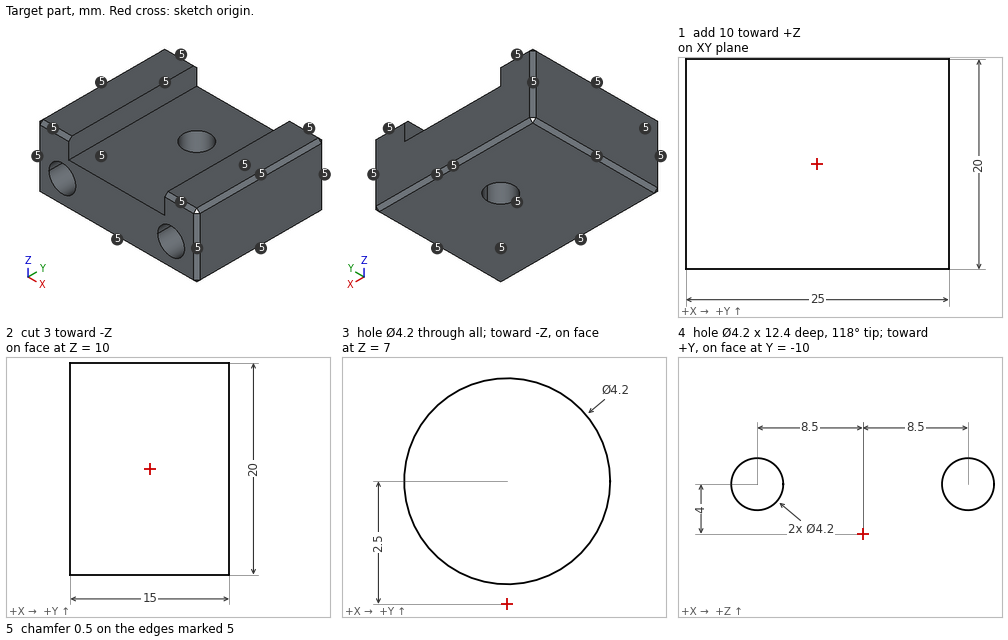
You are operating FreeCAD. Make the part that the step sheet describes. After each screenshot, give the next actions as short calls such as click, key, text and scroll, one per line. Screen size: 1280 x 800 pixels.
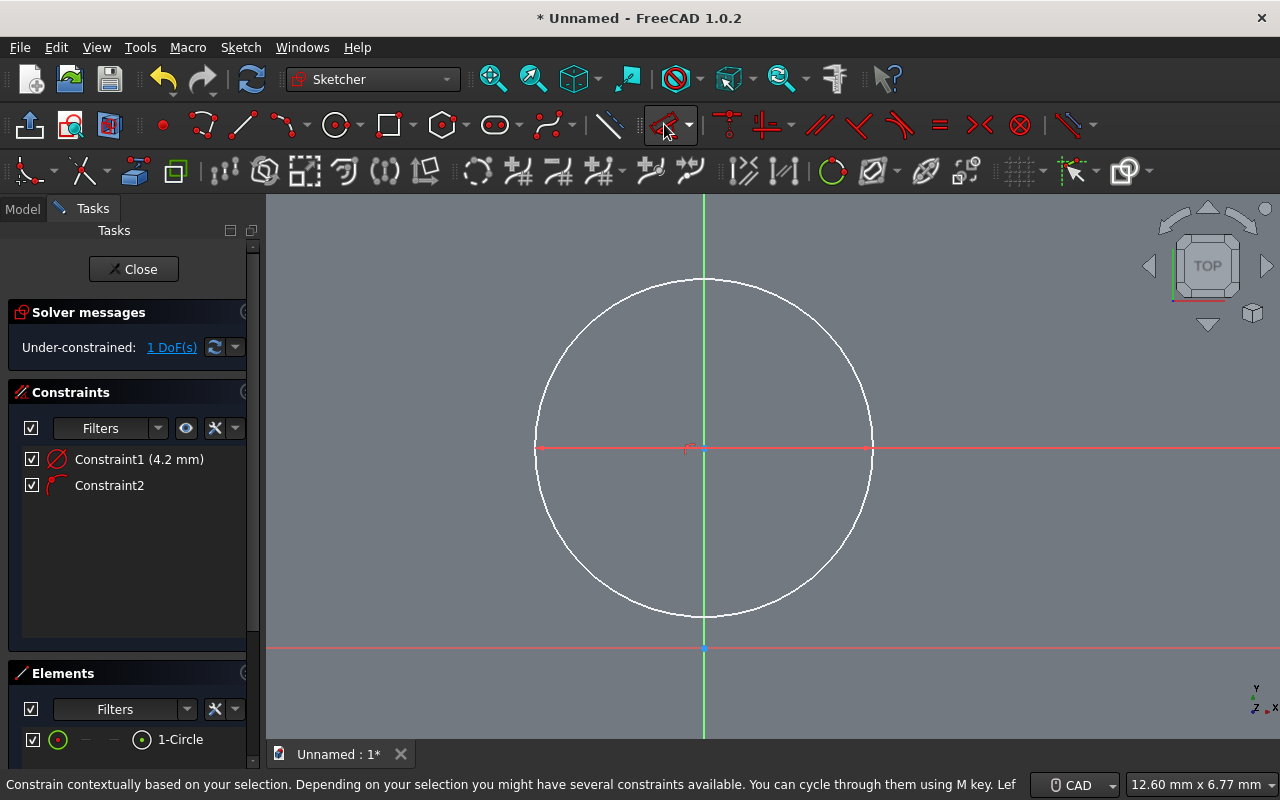
click(704, 448)
click(738, 548)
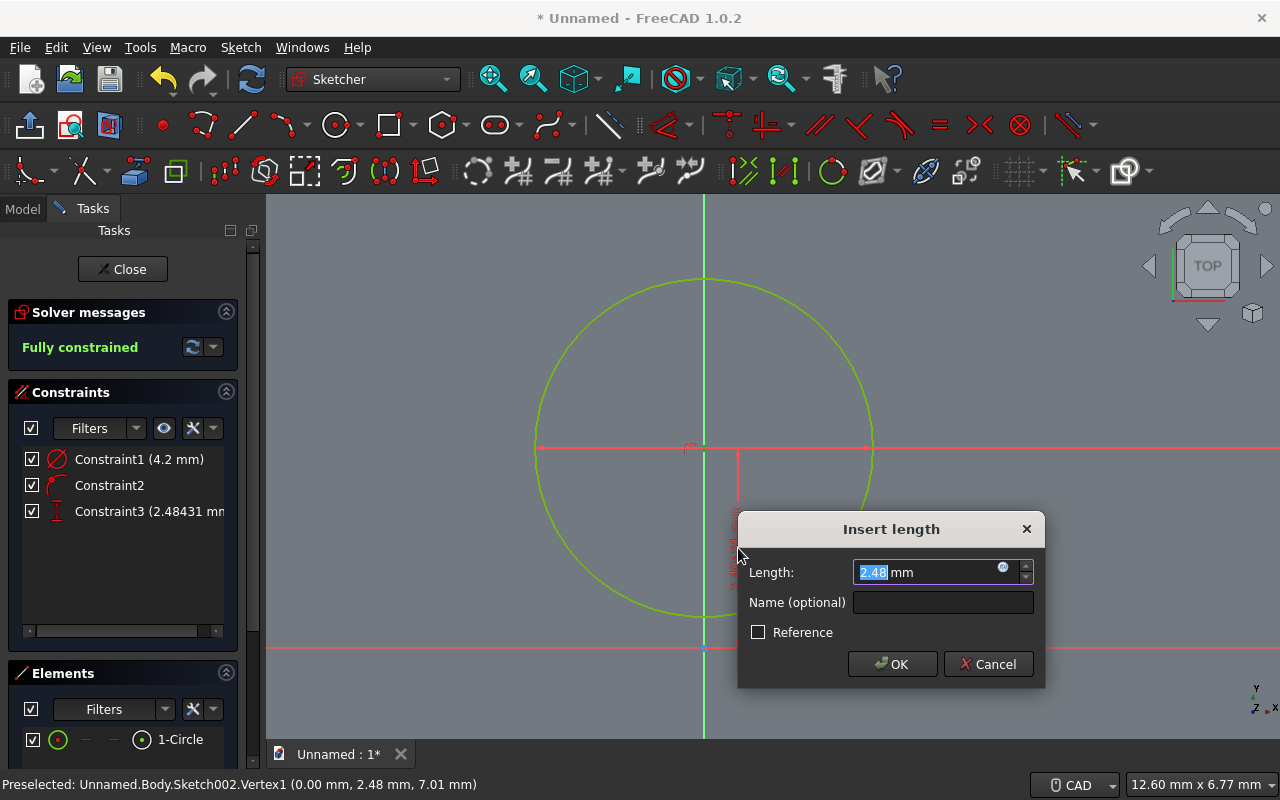
text(2.5)
key(Return)
key(Escape)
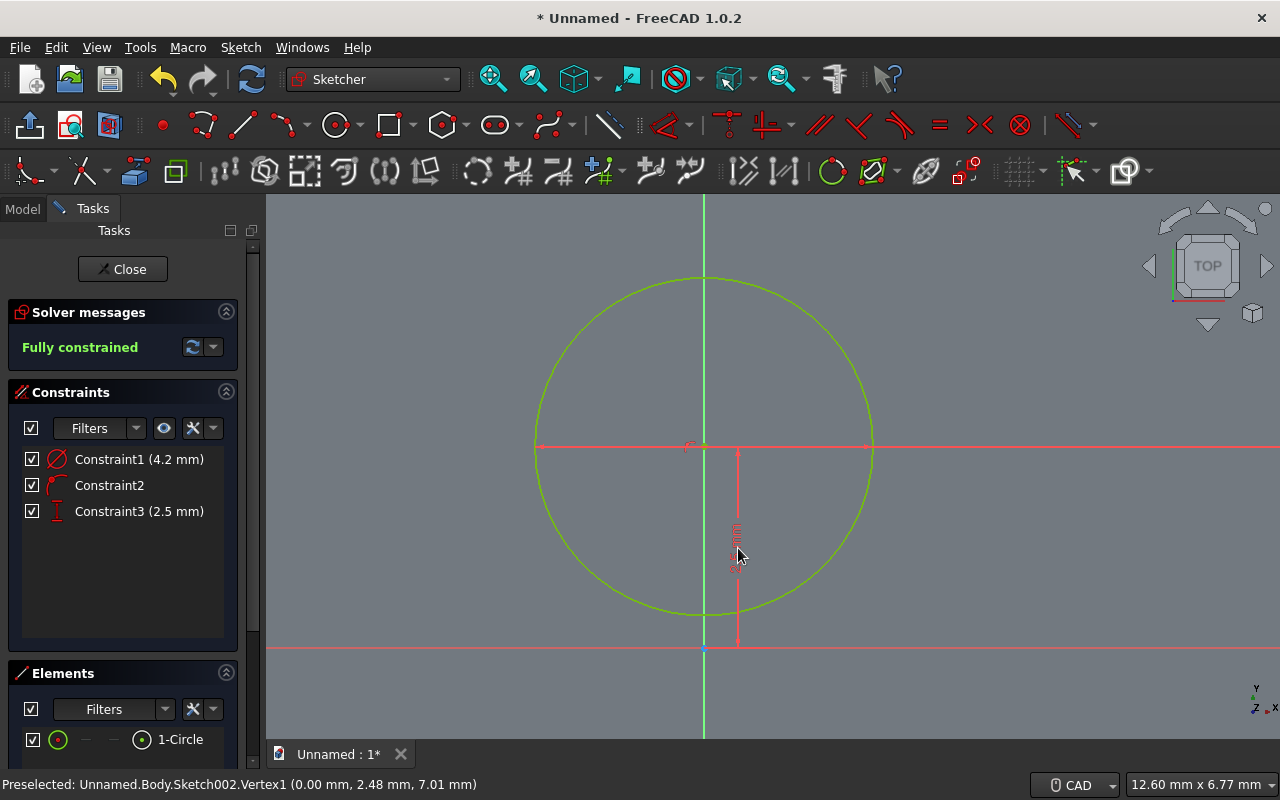
click(123, 269)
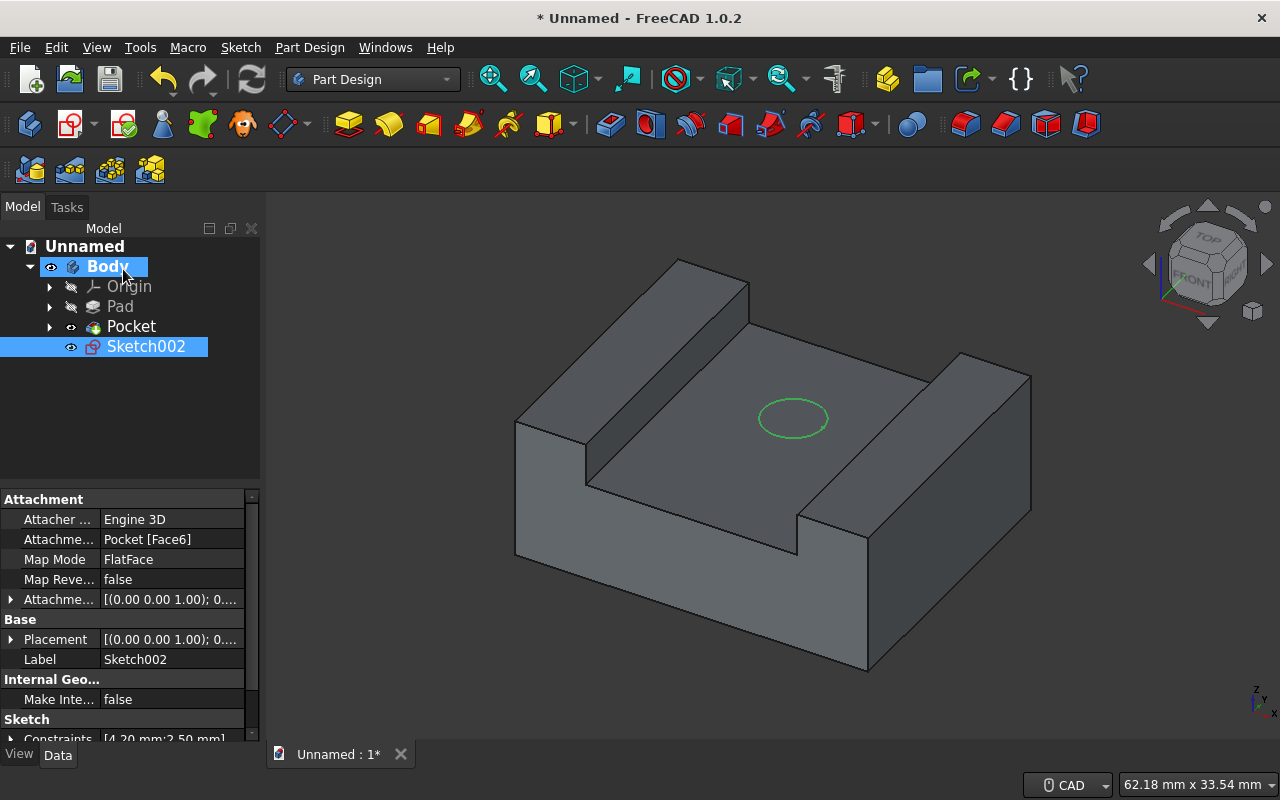
click(652, 124)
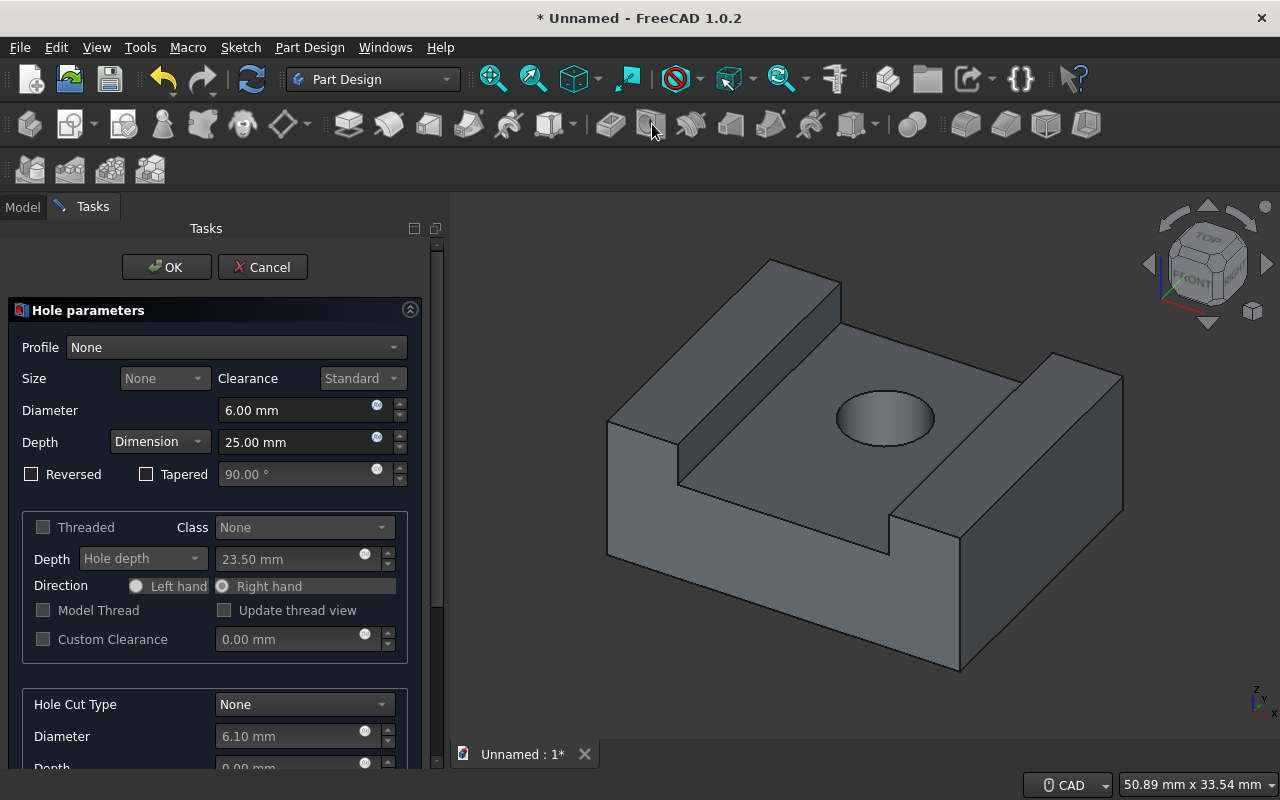
triple_click(305, 410)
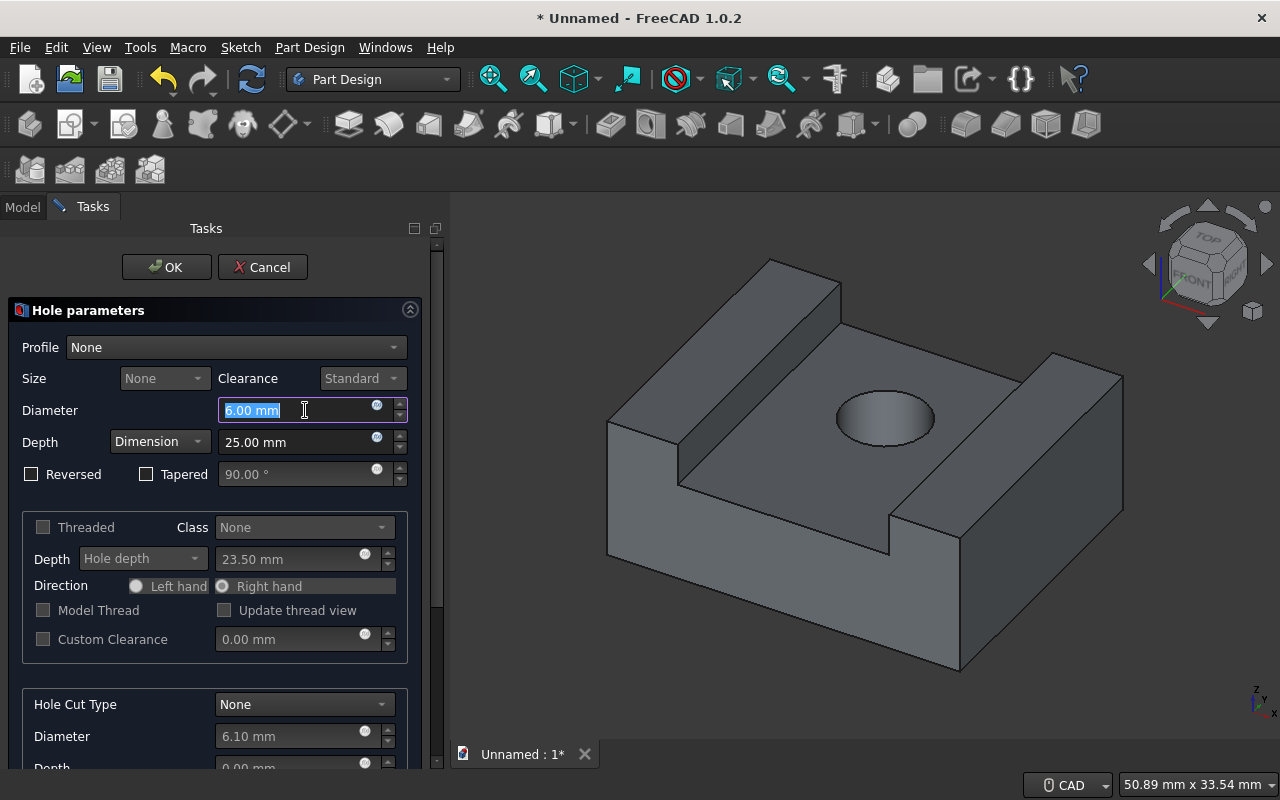
text(4.2)
key(Tab)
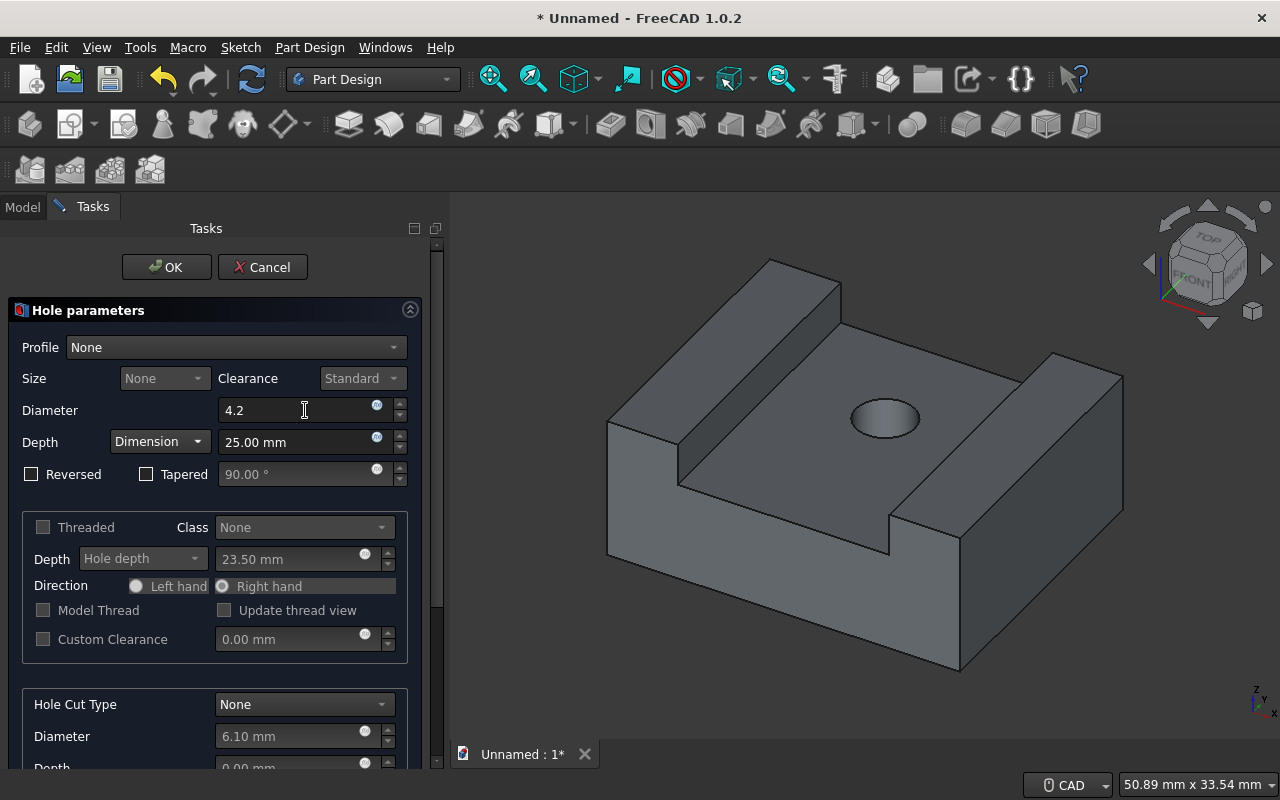
click(161, 442)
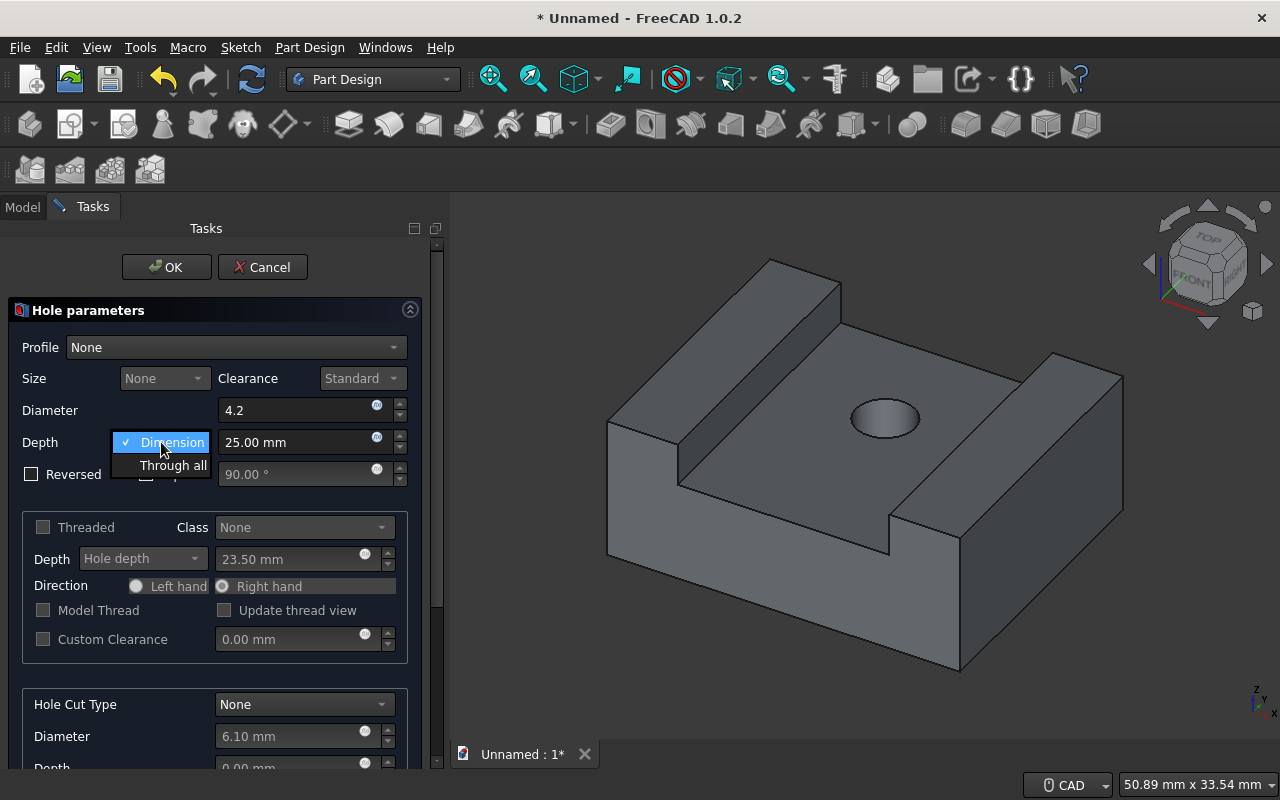
click(160, 466)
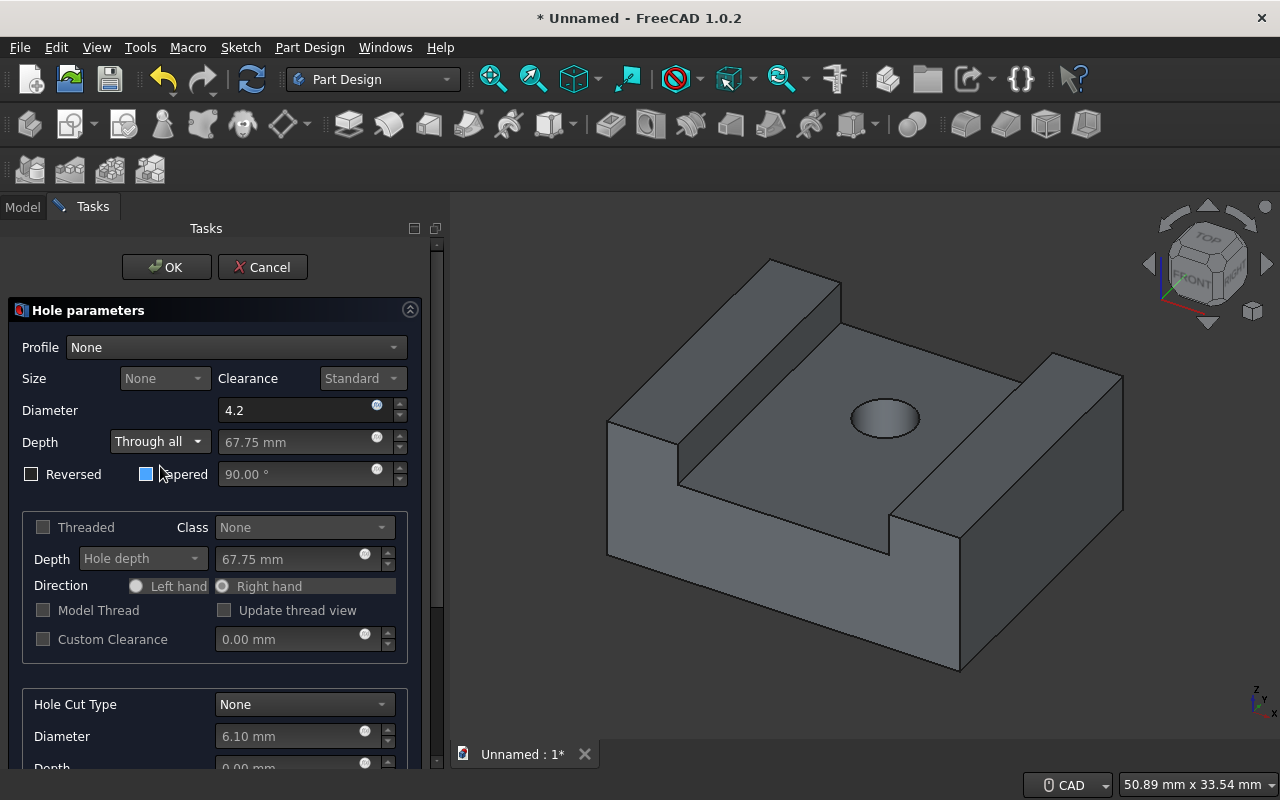
click(167, 267)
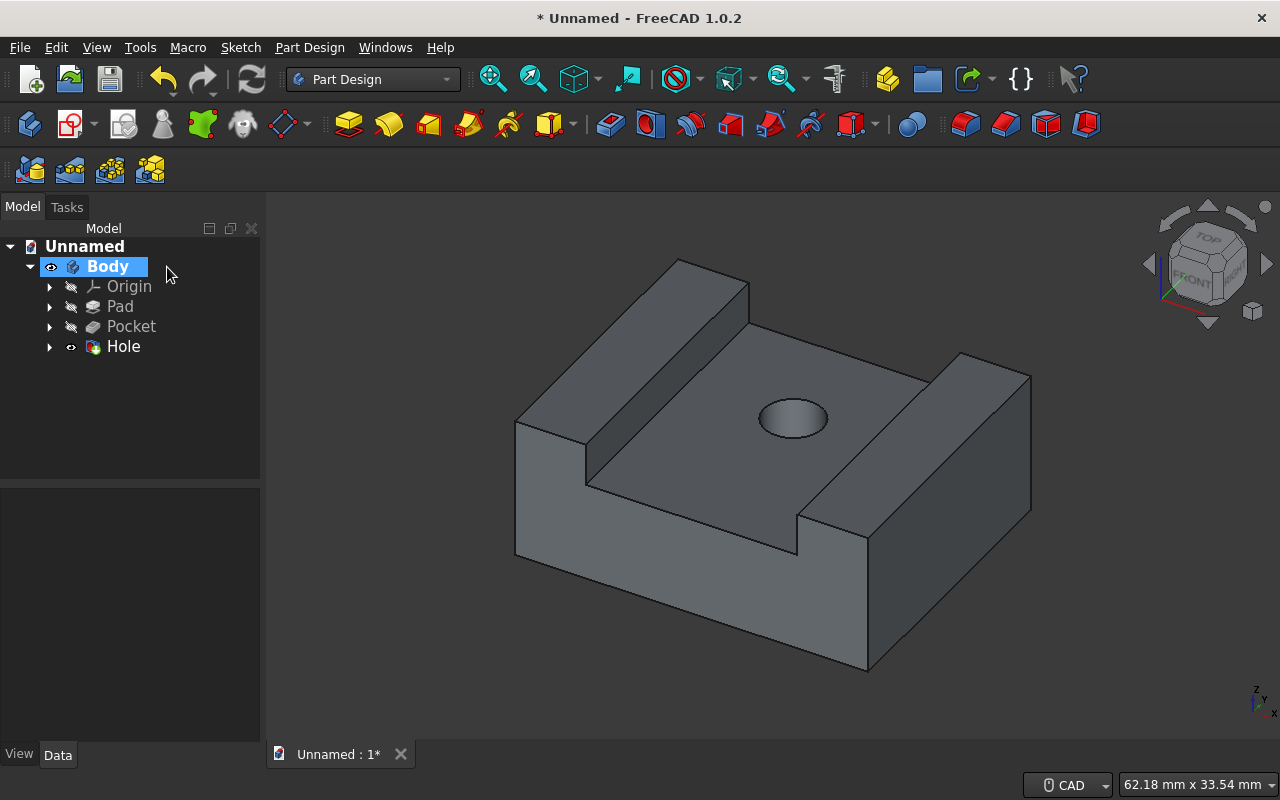
click(792, 598)